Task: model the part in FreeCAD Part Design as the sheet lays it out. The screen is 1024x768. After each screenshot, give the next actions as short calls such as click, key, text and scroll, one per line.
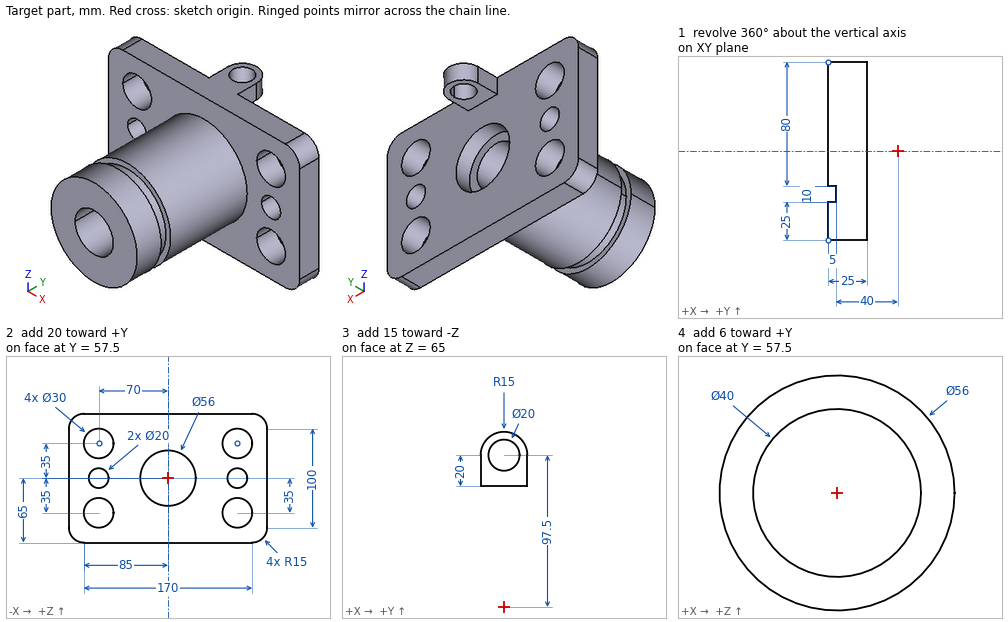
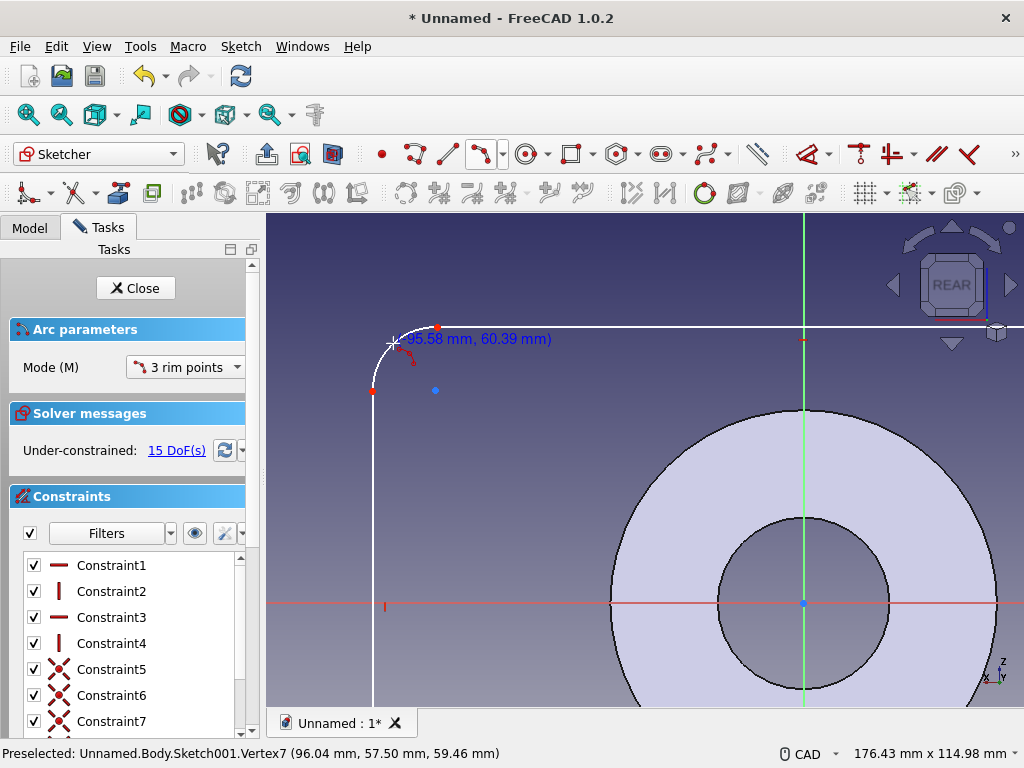
scroll(391, 343, down, 4)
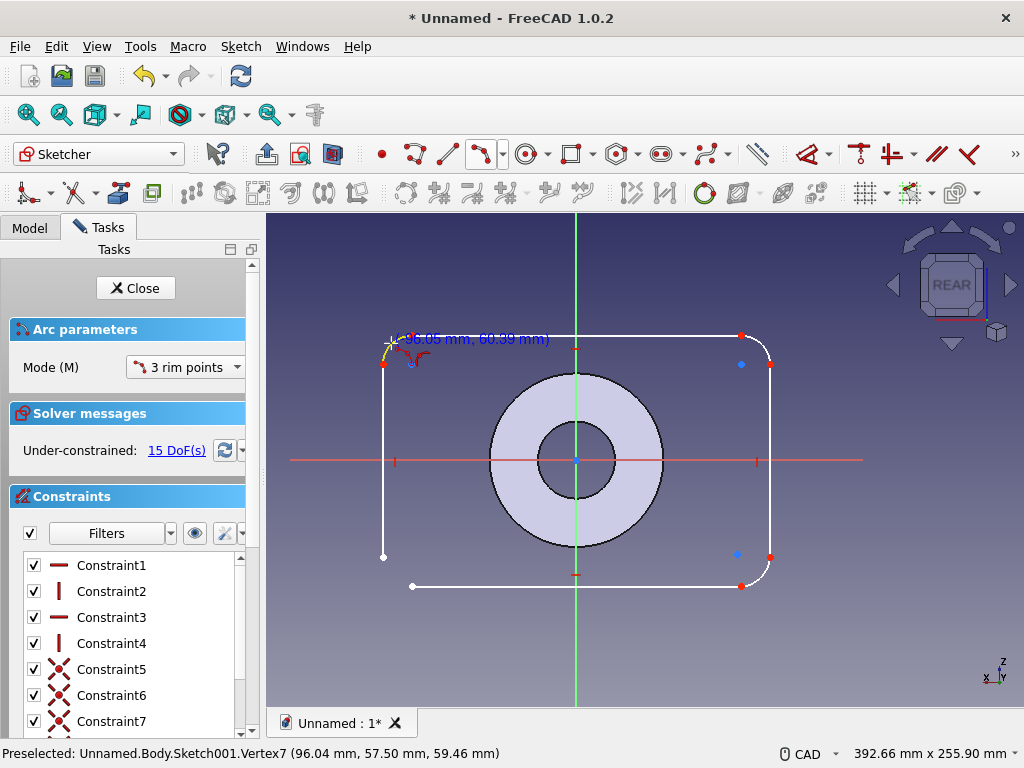
click(383, 558)
click(412, 587)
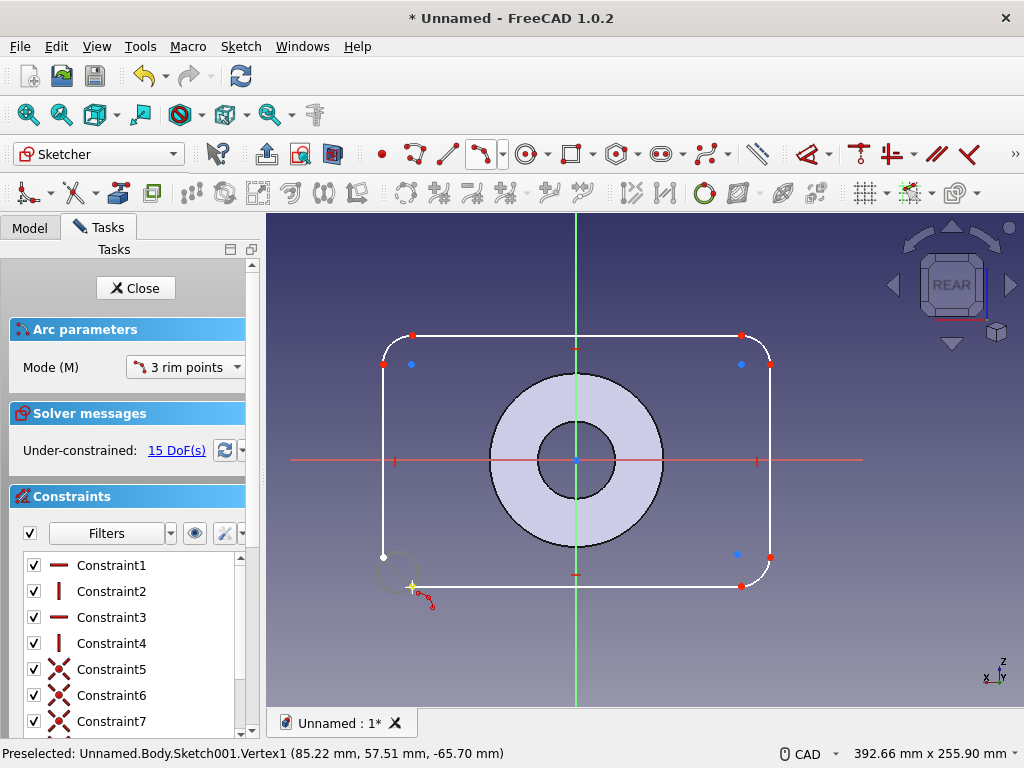
scroll(392, 577, up, 4)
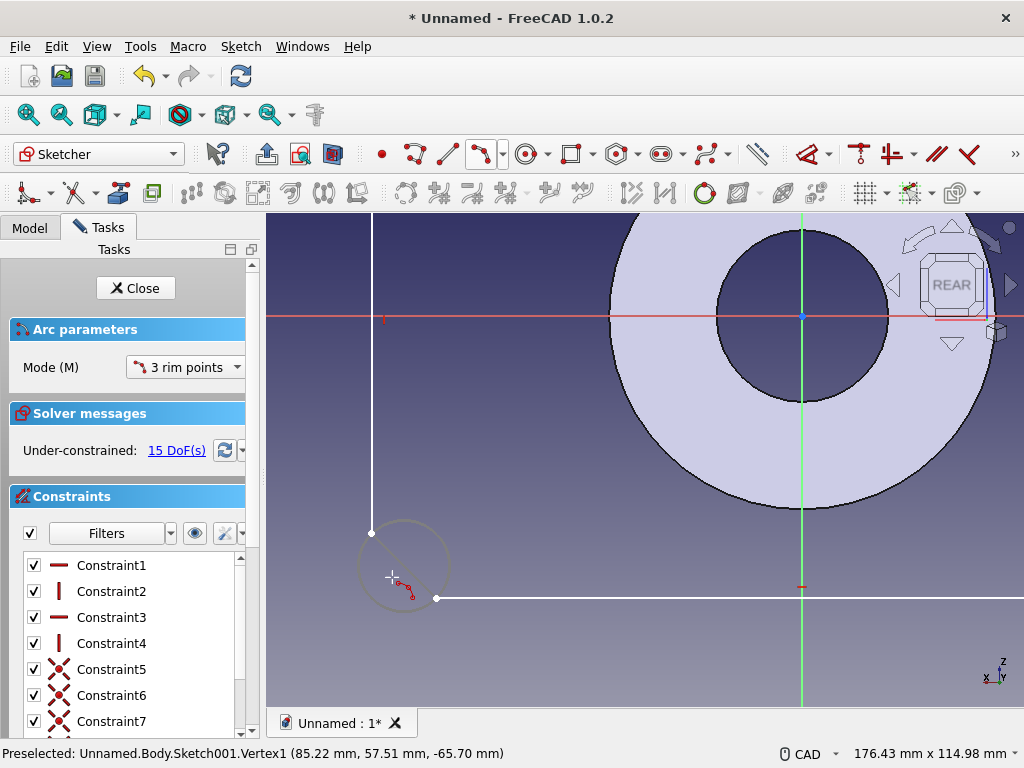
click(392, 576)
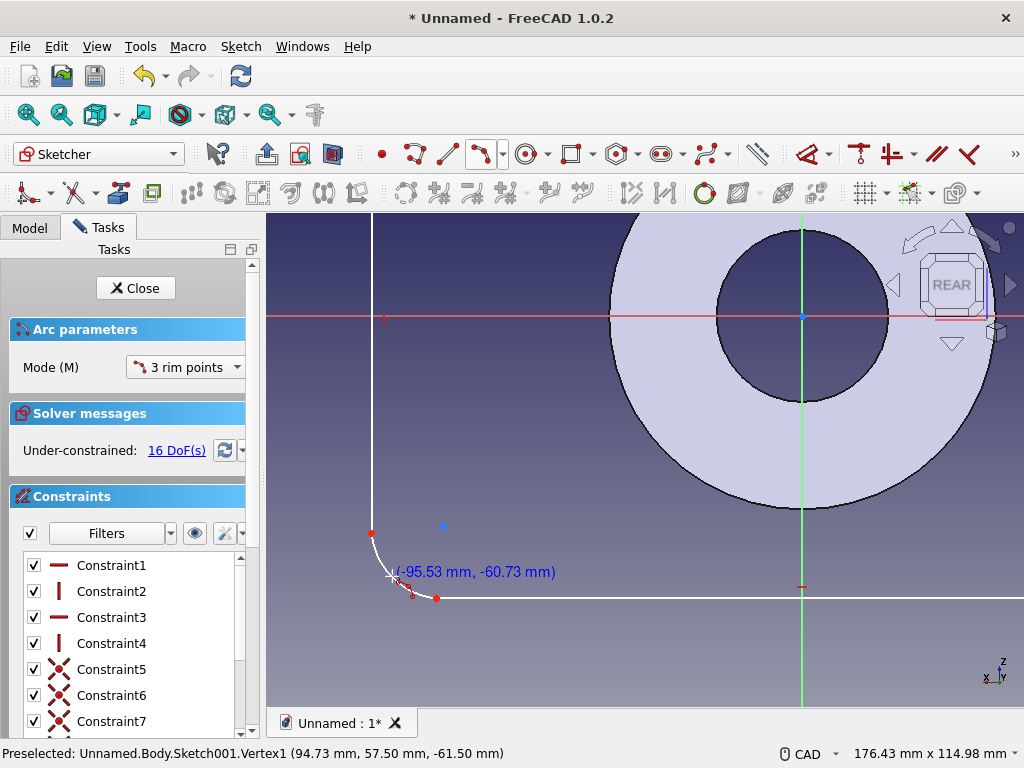
click(526, 154)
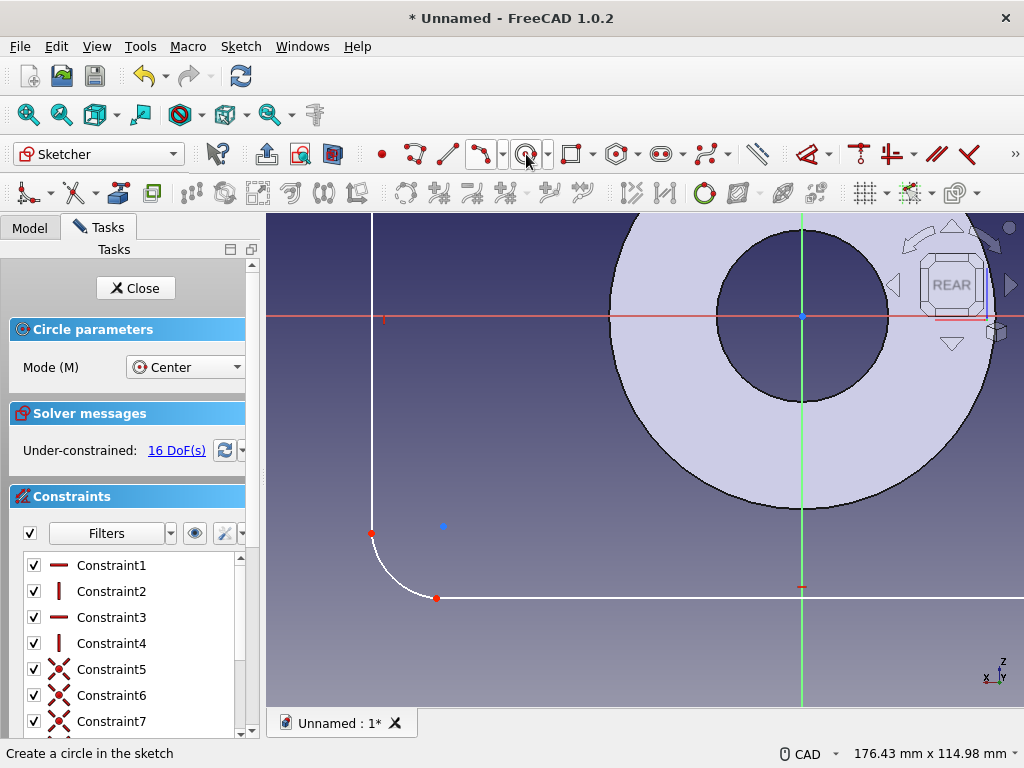
scroll(392, 577, down, 4)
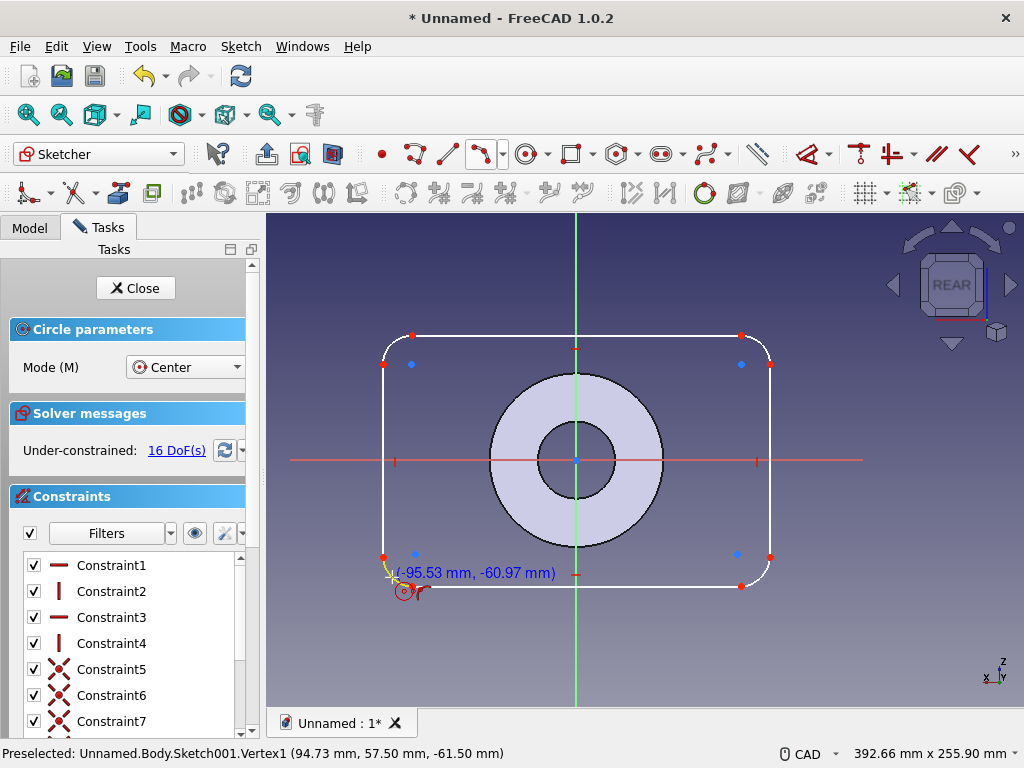
click(441, 393)
move(462, 372)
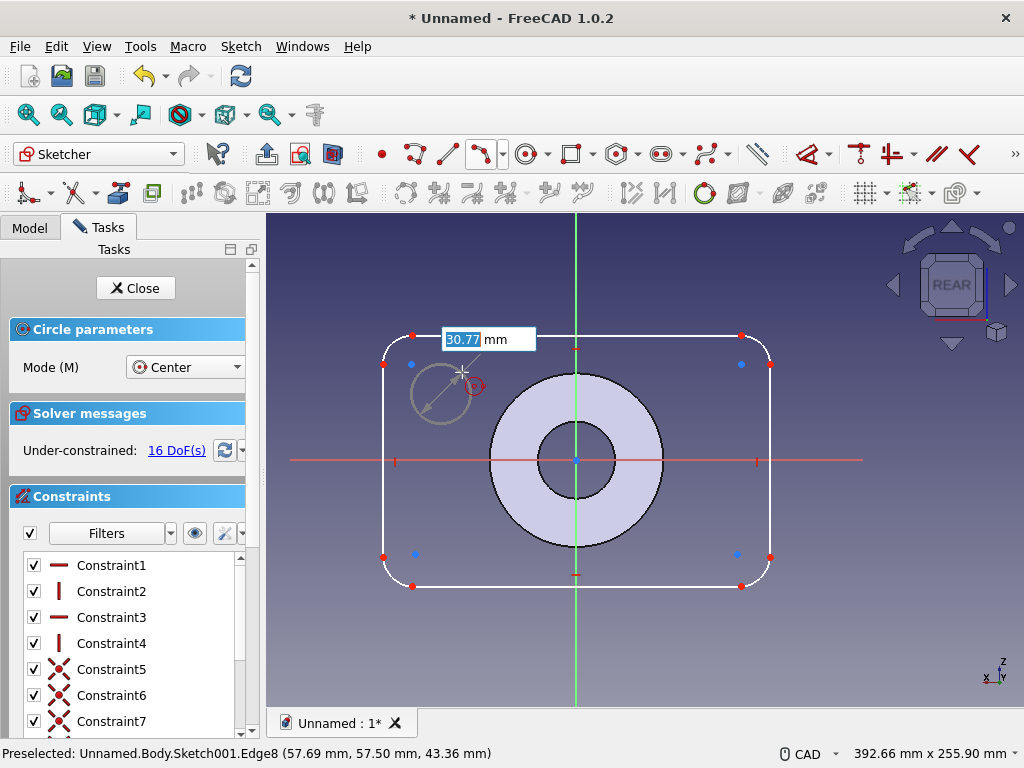
text(30)
key(Return)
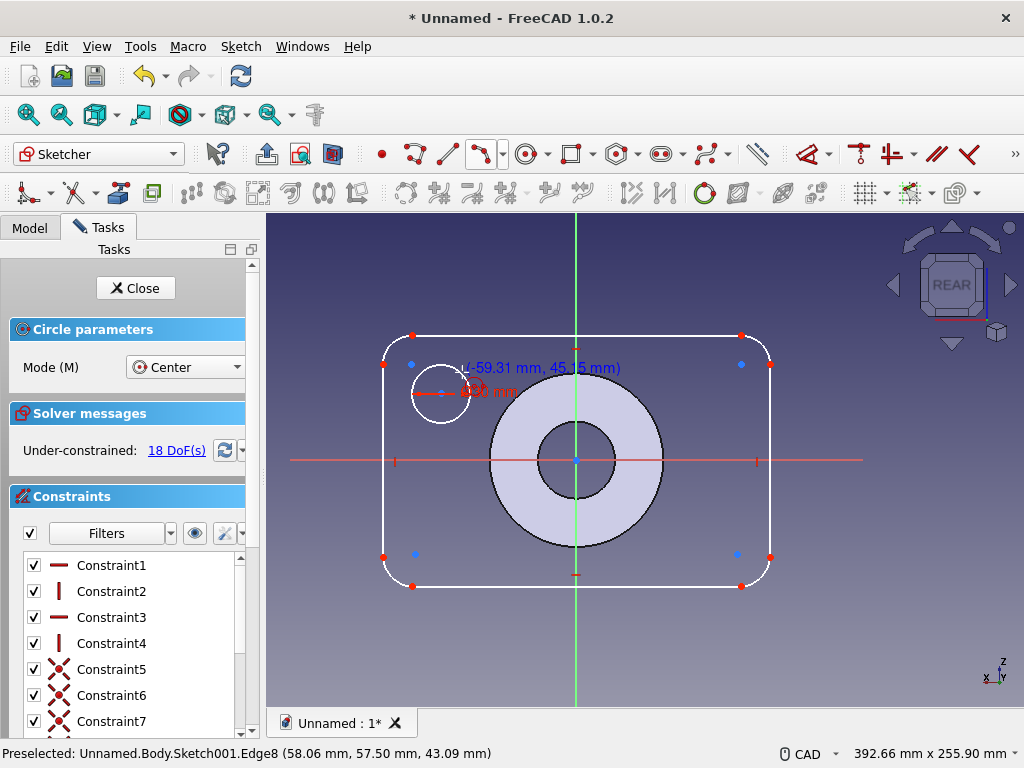
click(712, 393)
move(691, 372)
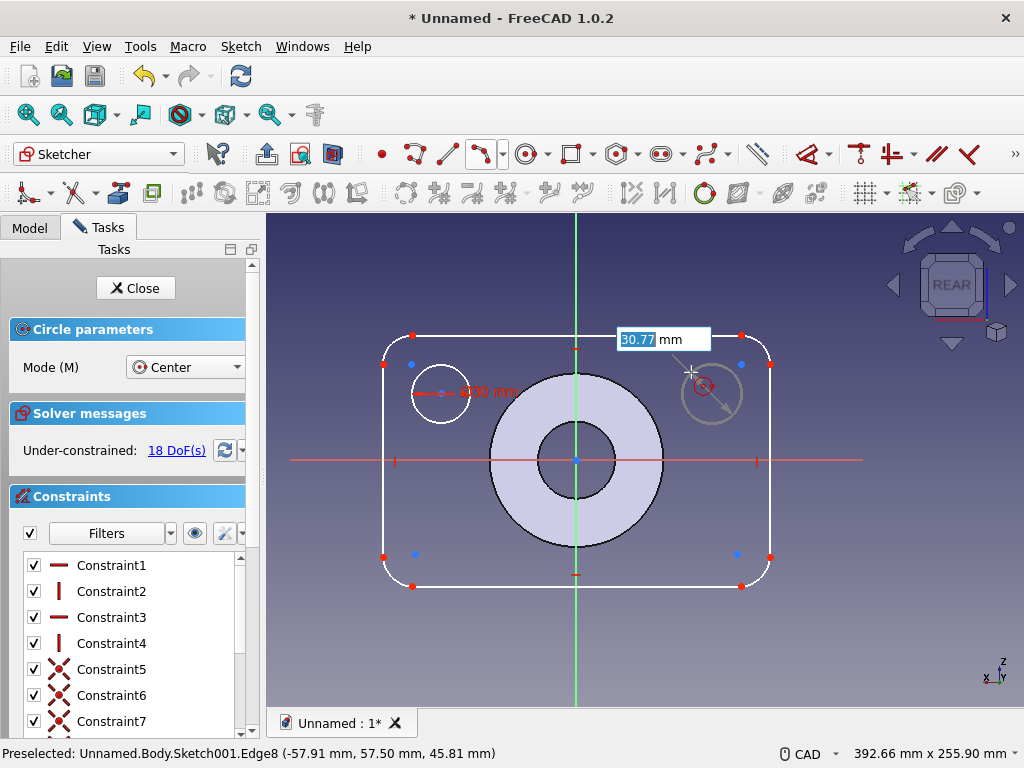
text(30)
key(Return)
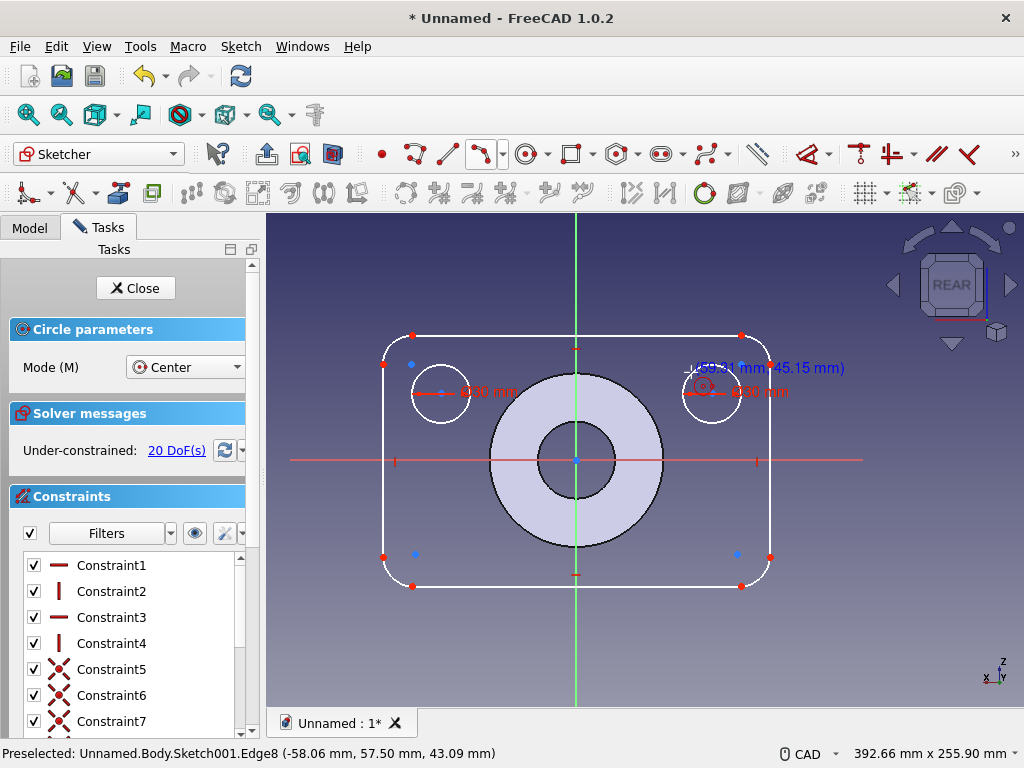
click(441, 460)
move(448, 442)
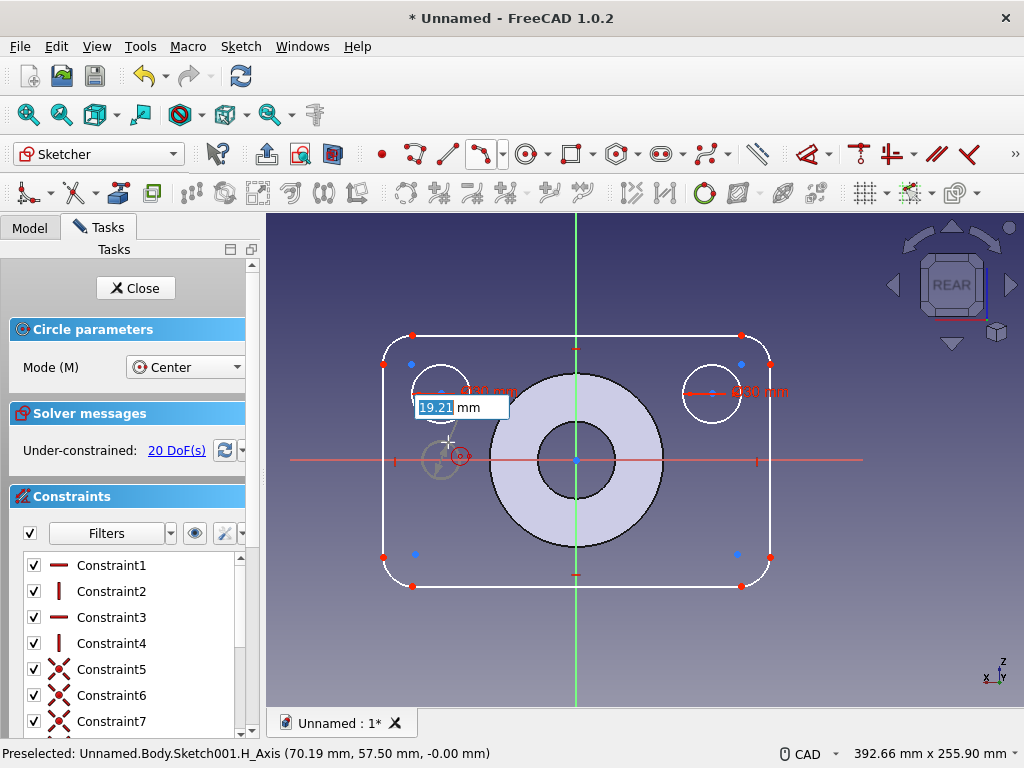
text(20)
key(Return)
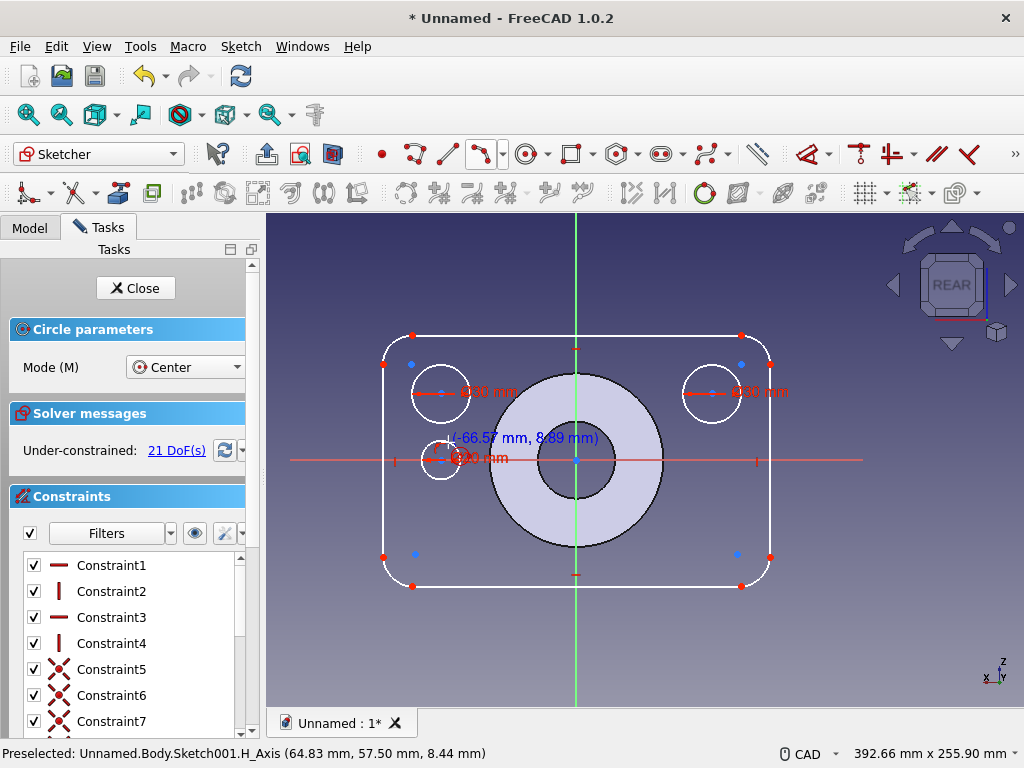
click(441, 528)
move(462, 507)